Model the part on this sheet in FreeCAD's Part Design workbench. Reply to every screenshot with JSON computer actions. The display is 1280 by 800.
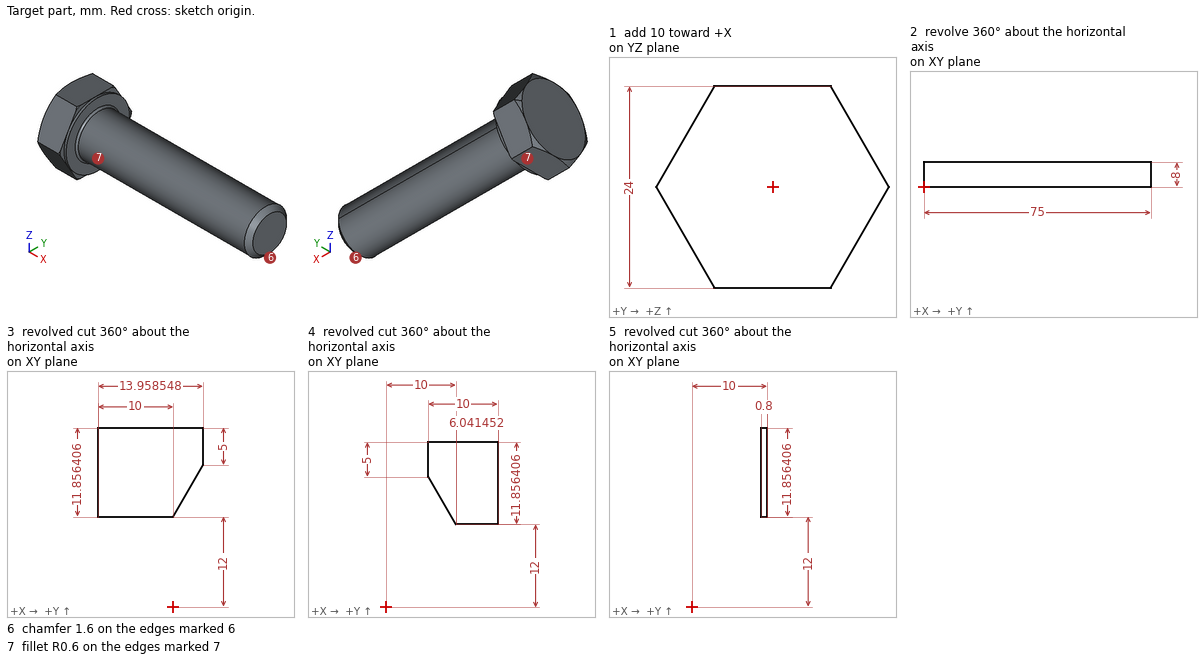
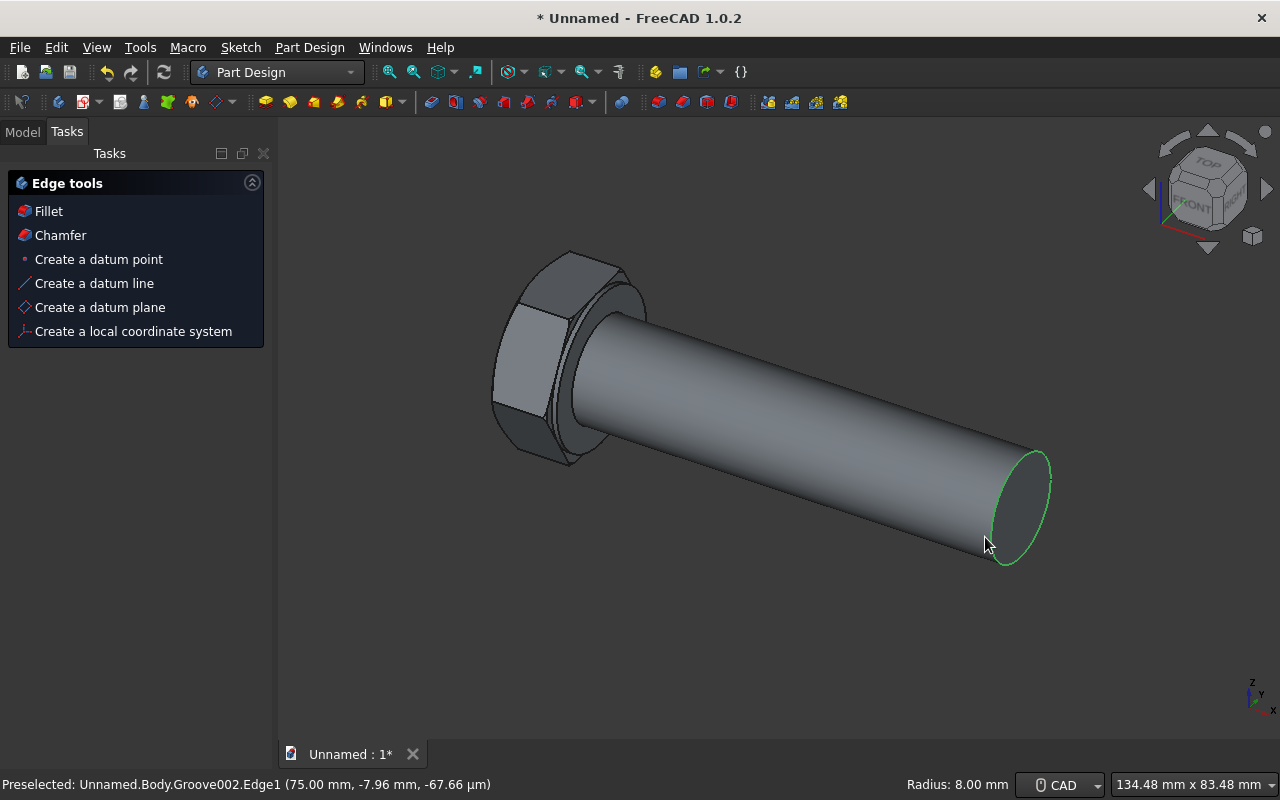
{"action": "left_click", "coordinate": [684, 102]}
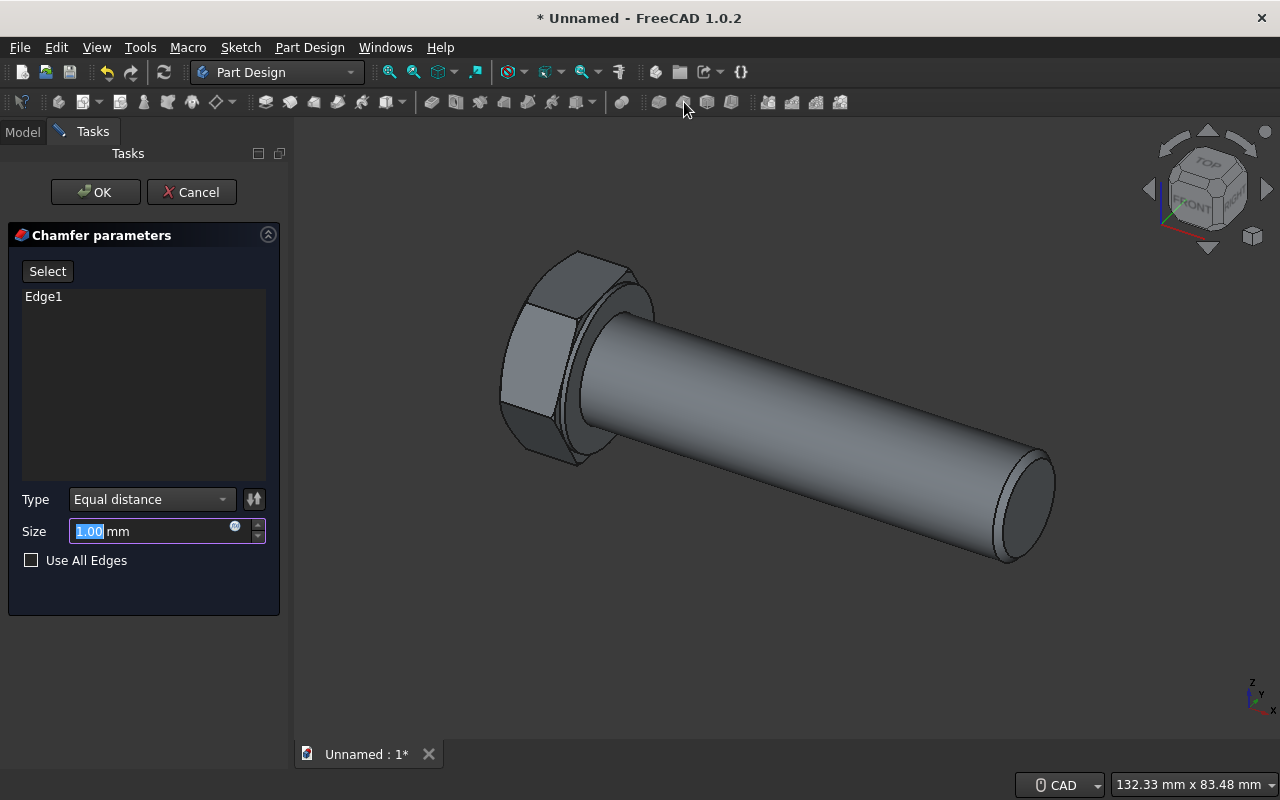
{"action": "type", "text": "1.6"}
{"action": "key", "text": "Tab"}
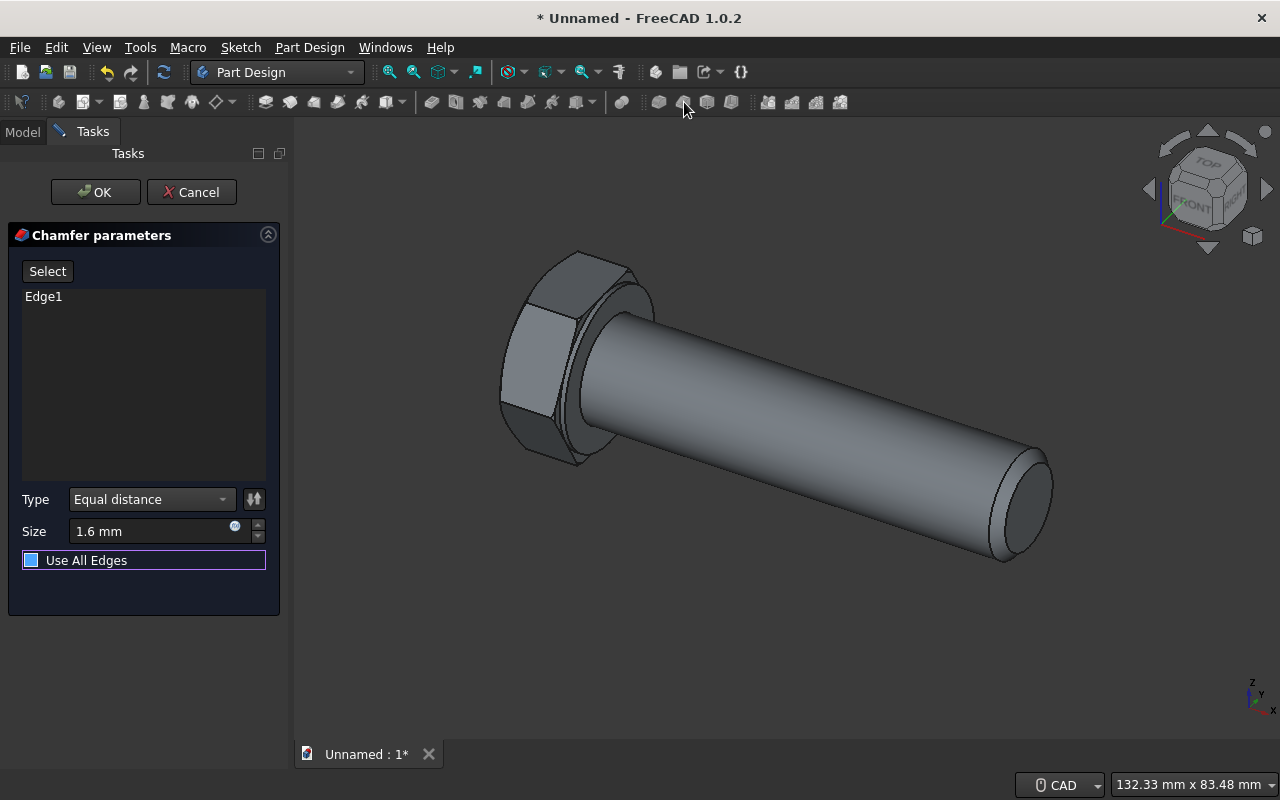
{"action": "left_click", "coordinate": [96, 192]}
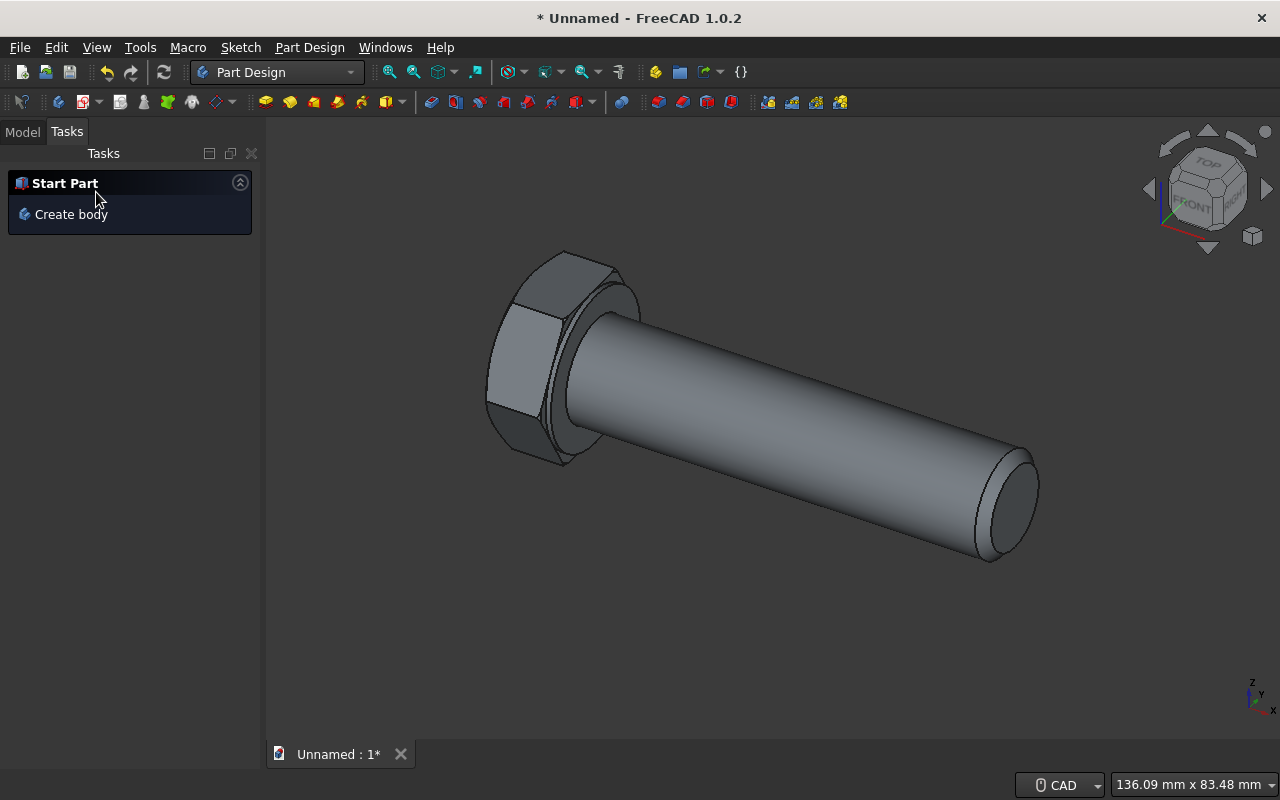
{"action": "key", "text": "0"}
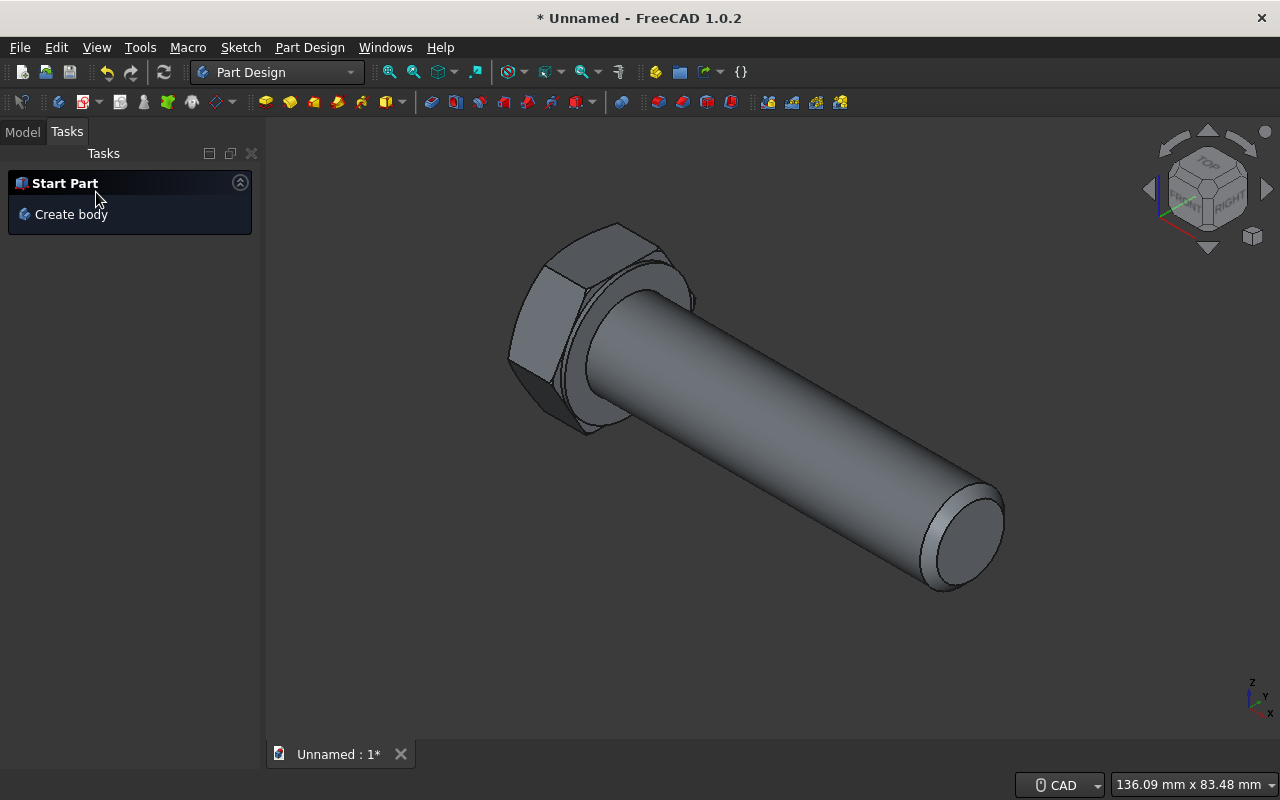
{"action": "key", "text": "2"}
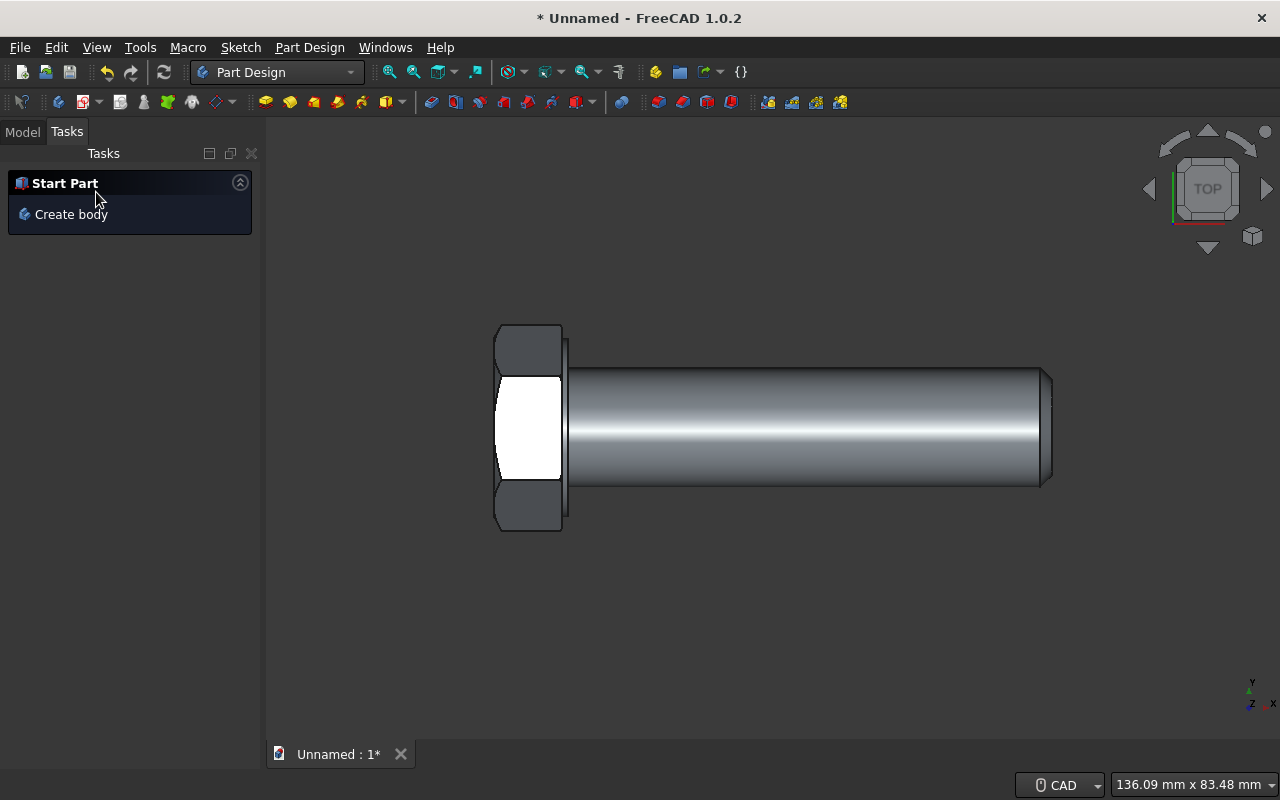
{"action": "key", "text": "1"}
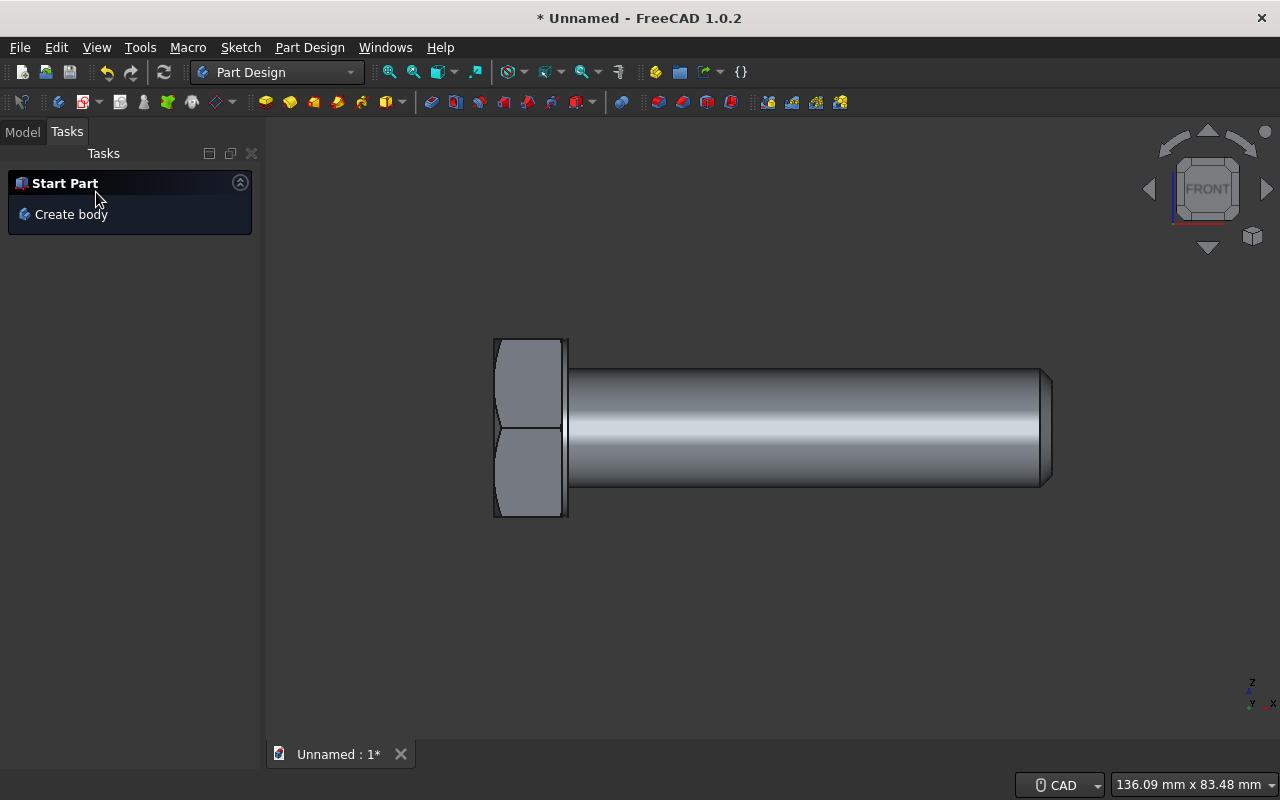
{"action": "key", "text": "3"}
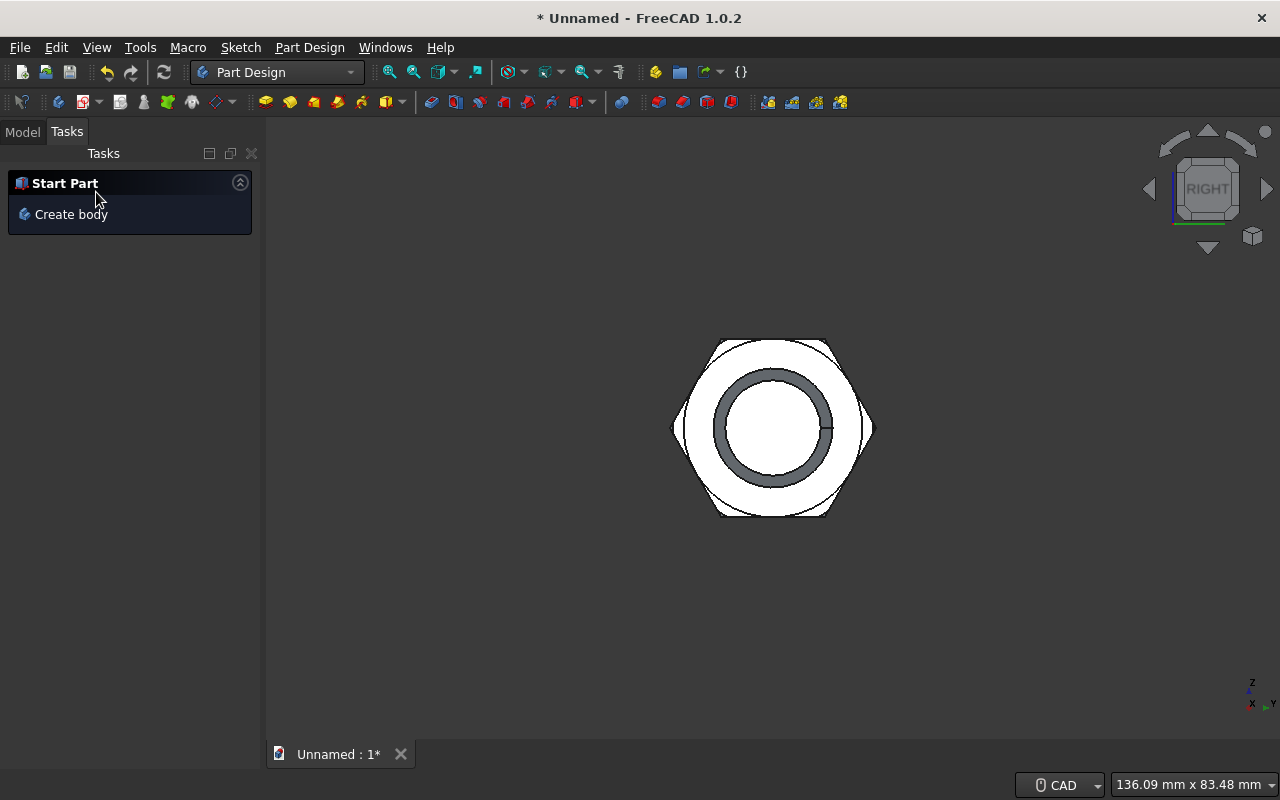
{"action": "left_click", "coordinate": [390, 72]}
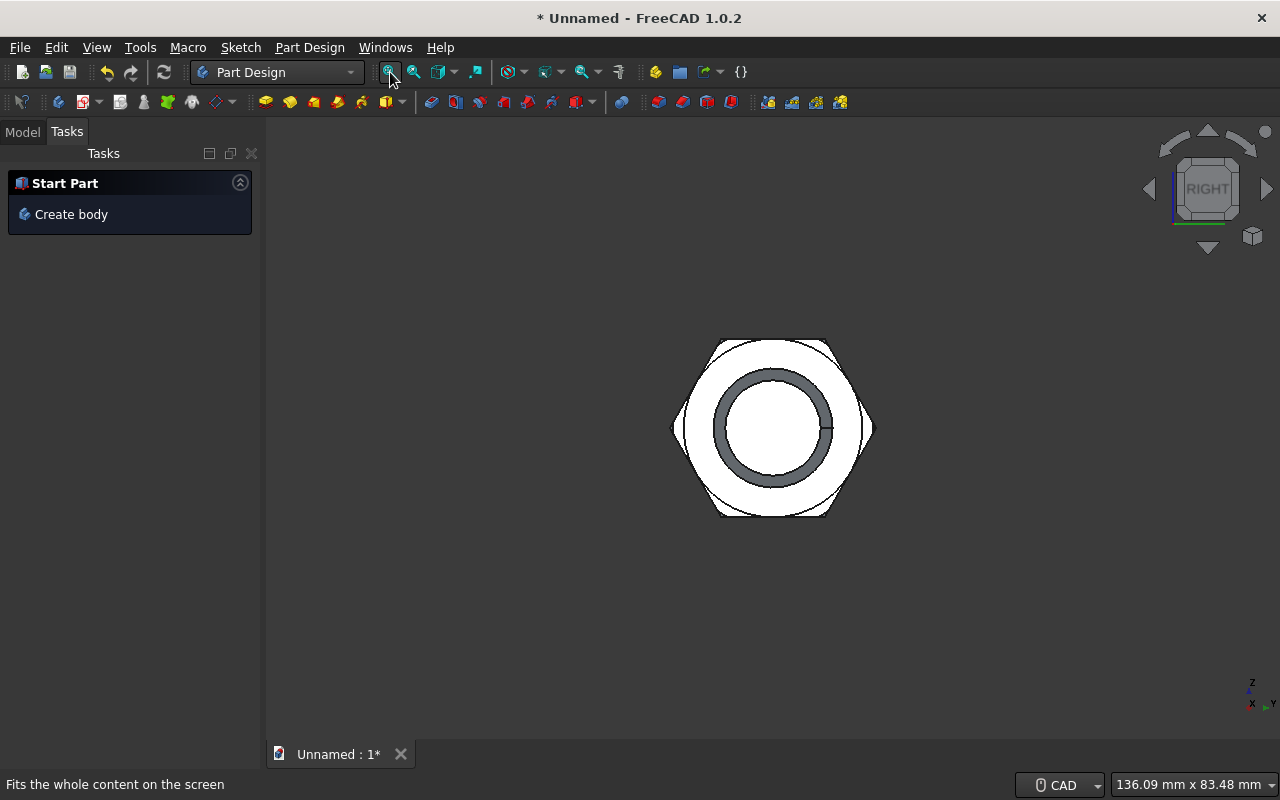
{"action": "key", "text": "5"}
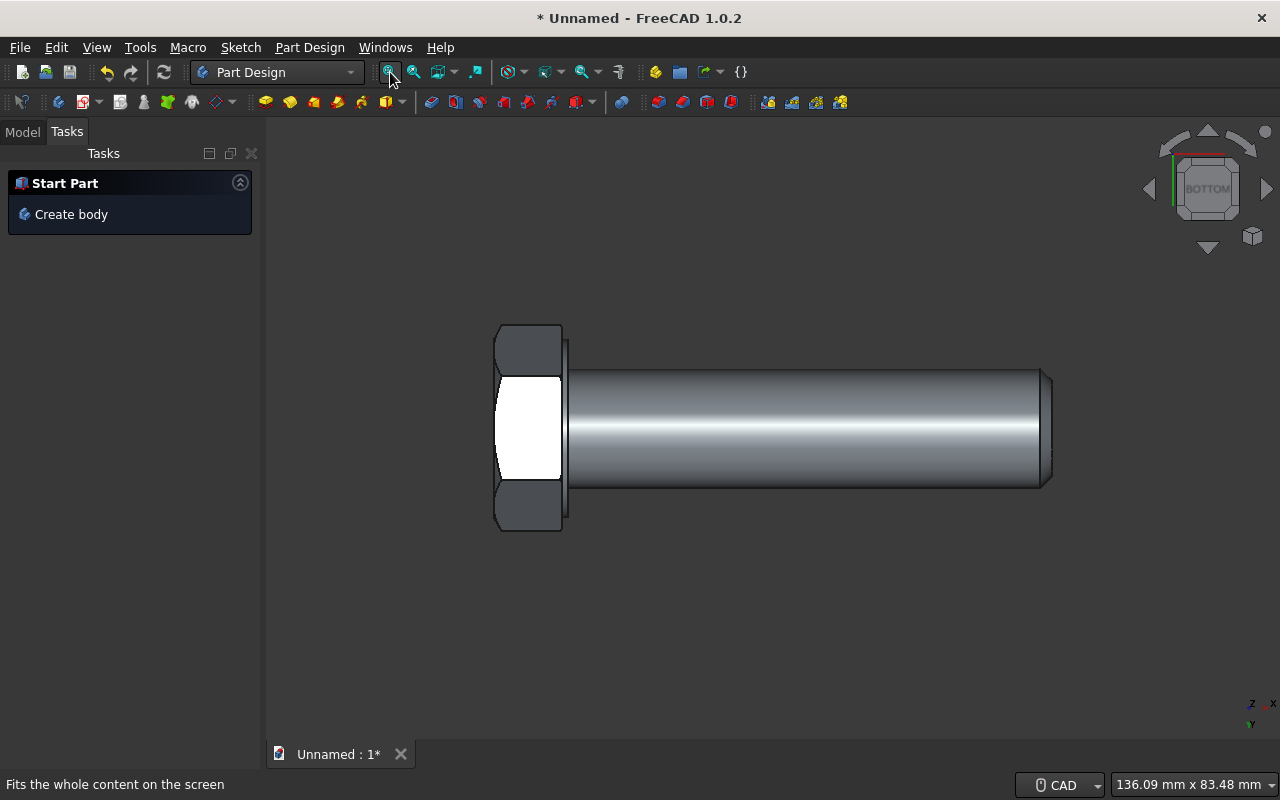
{"action": "key", "text": "4"}